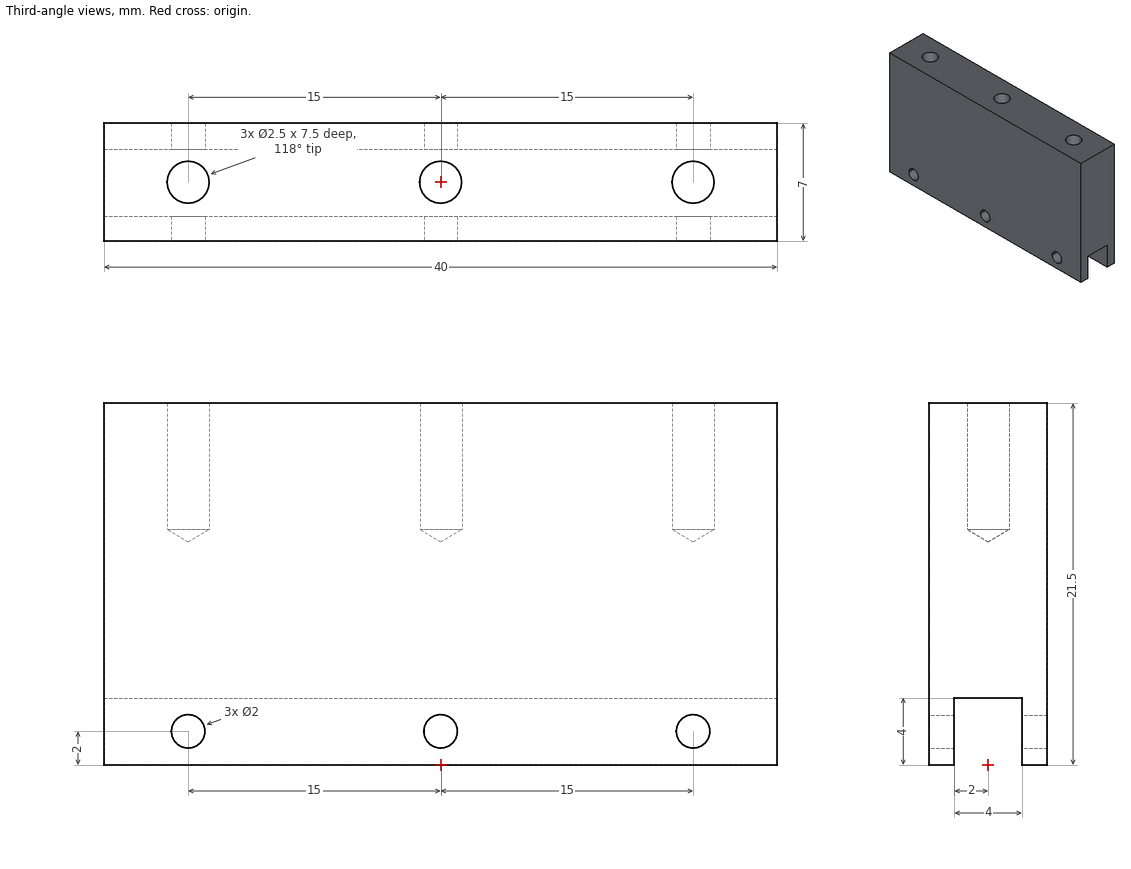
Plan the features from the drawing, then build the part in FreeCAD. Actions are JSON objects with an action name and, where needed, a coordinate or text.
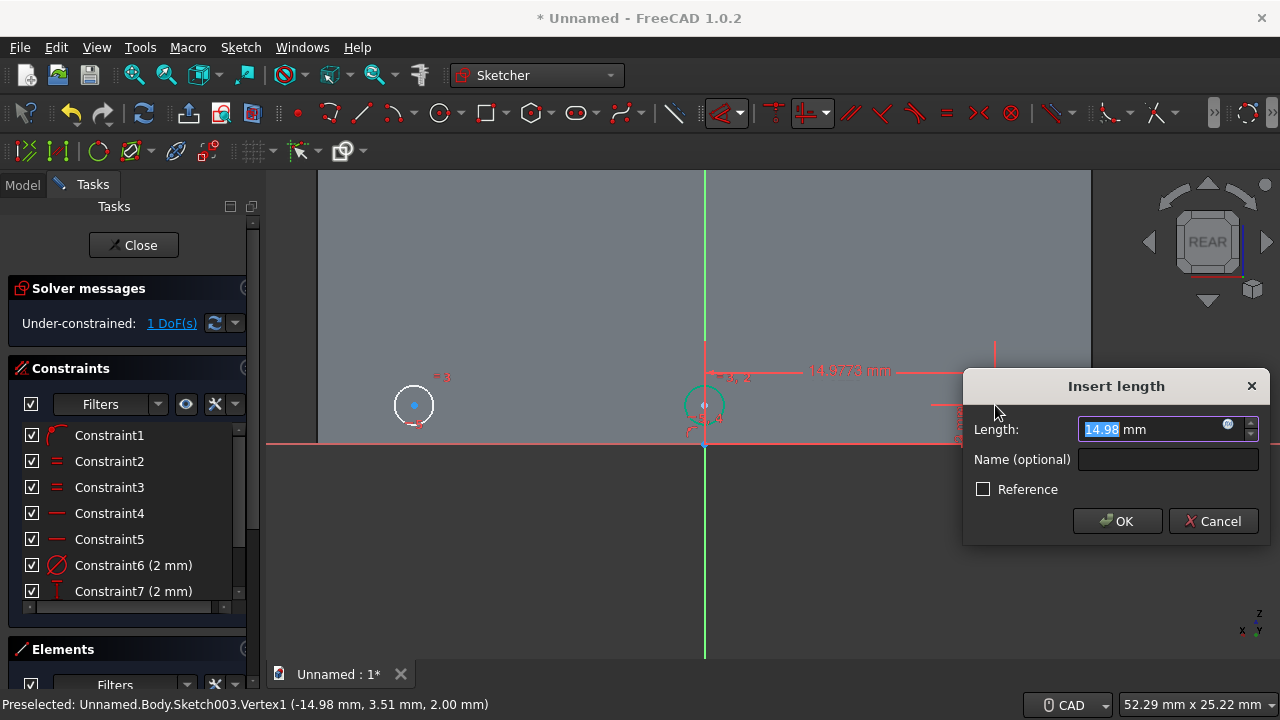
{"action": "type", "text": "15"}
{"action": "key", "text": "Return"}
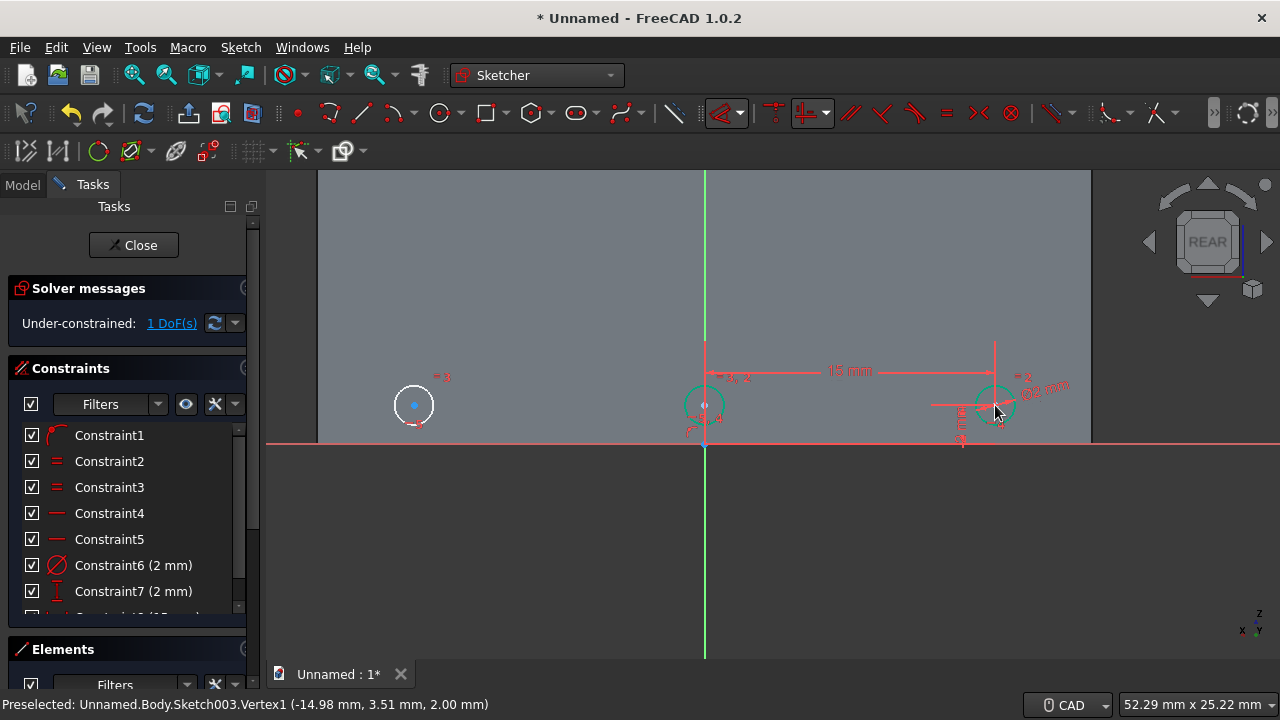
{"action": "left_click", "coordinate": [414, 405]}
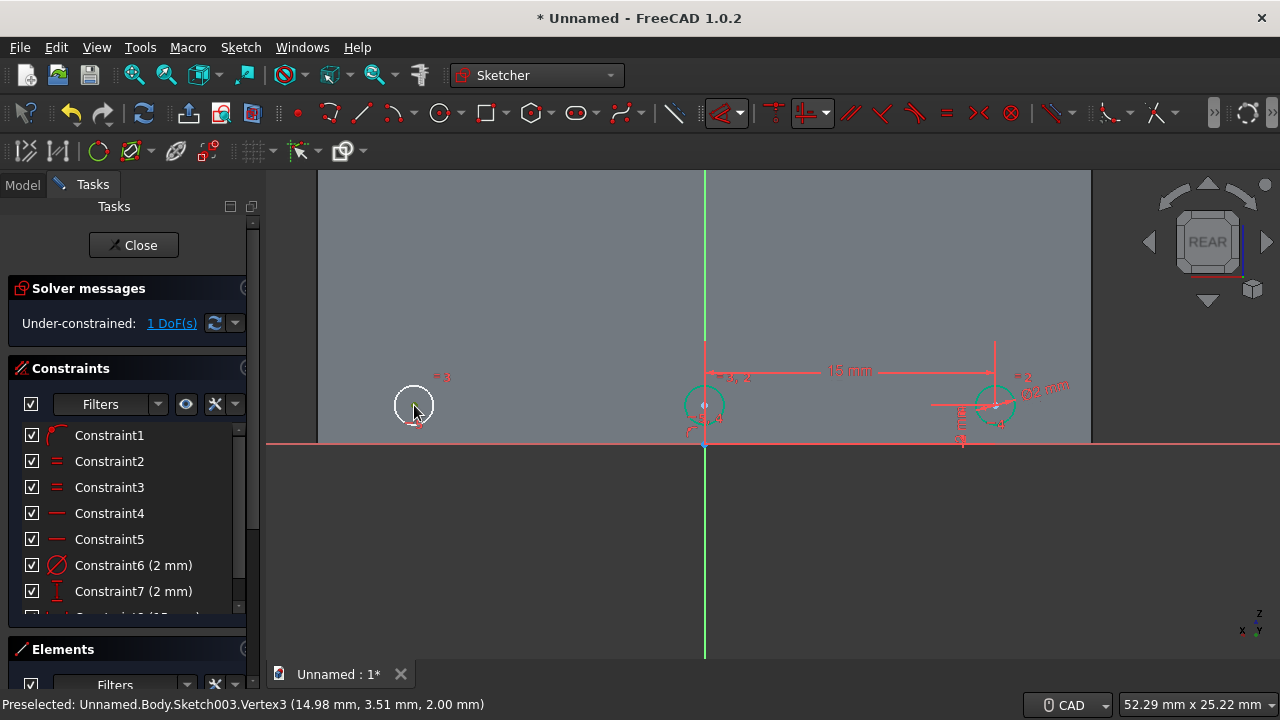
{"action": "left_click", "coordinate": [742, 114]}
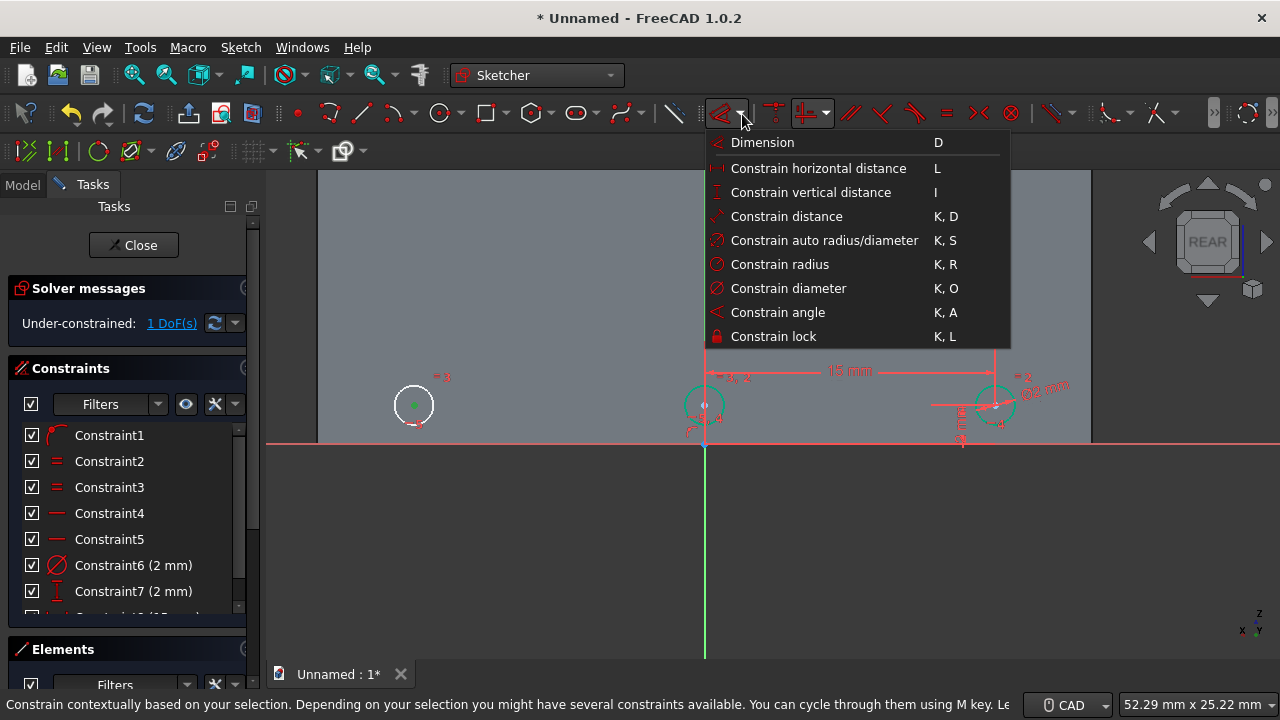
{"action": "left_click", "coordinate": [858, 168]}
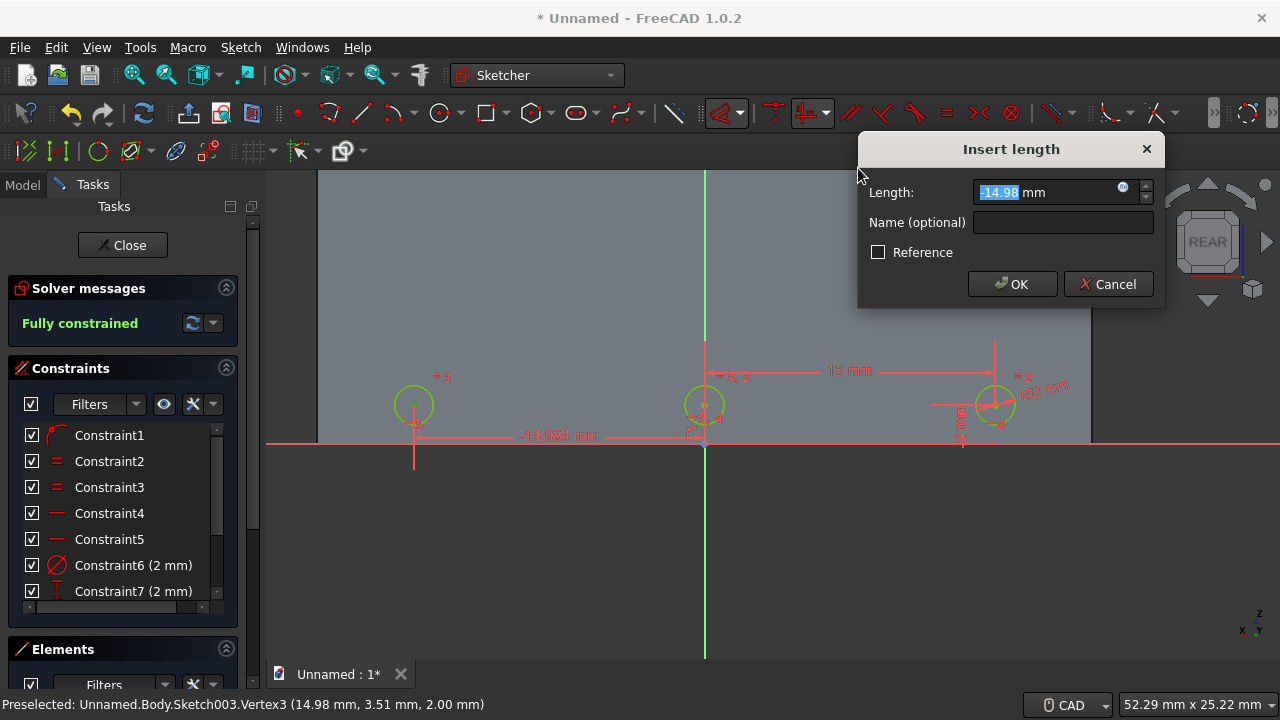
{"action": "type", "text": "-15"}
{"action": "key", "text": "Return"}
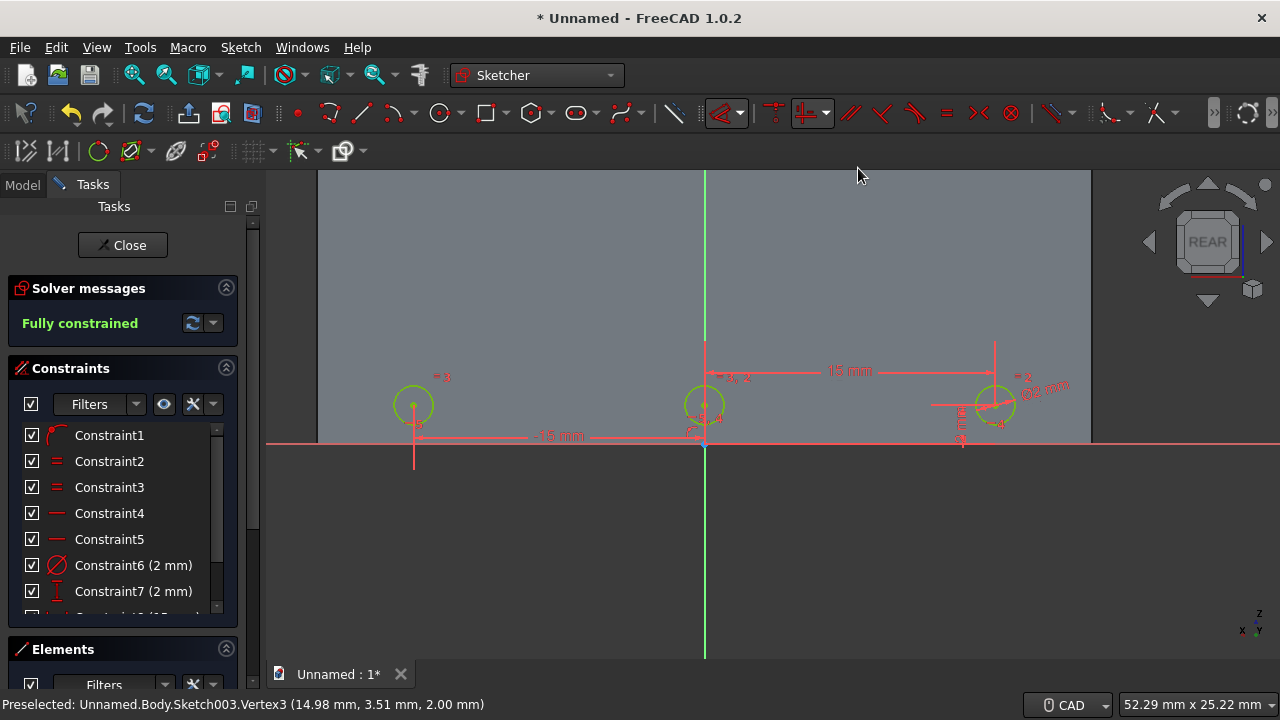
{"action": "left_click", "coordinate": [123, 245]}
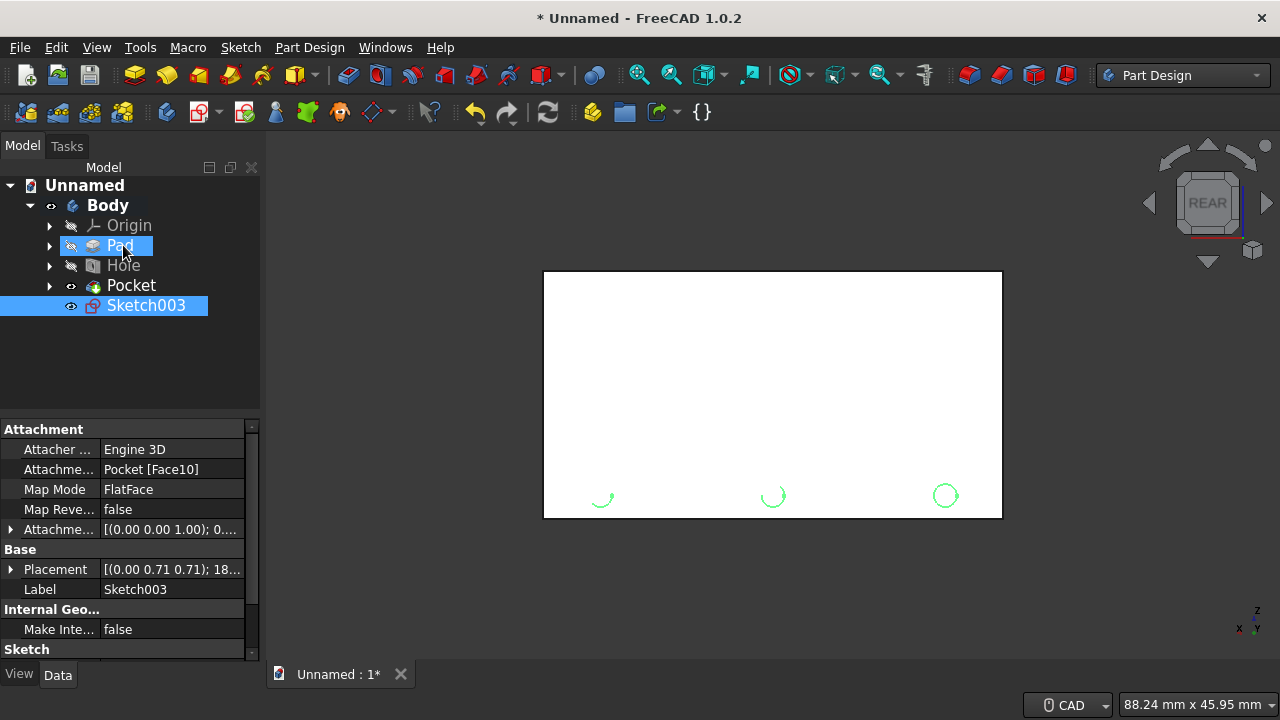
{"action": "left_click", "coordinate": [350, 76]}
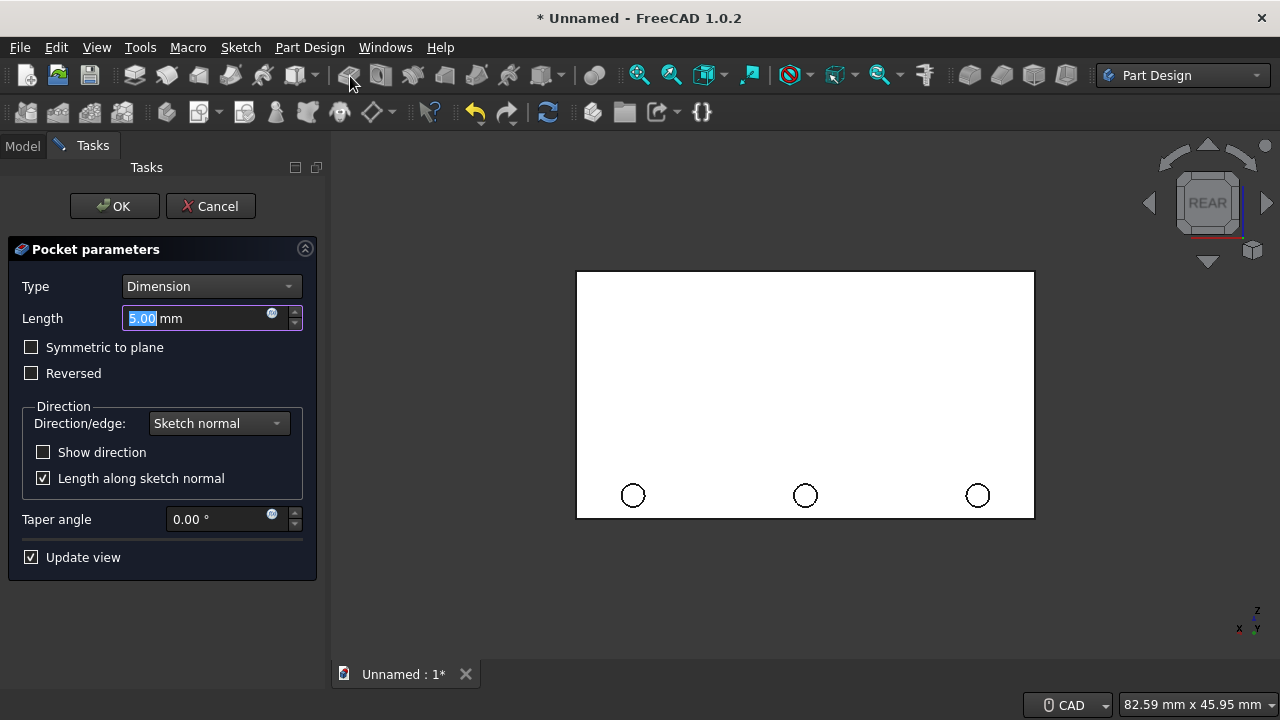
{"action": "left_click", "coordinate": [212, 286]}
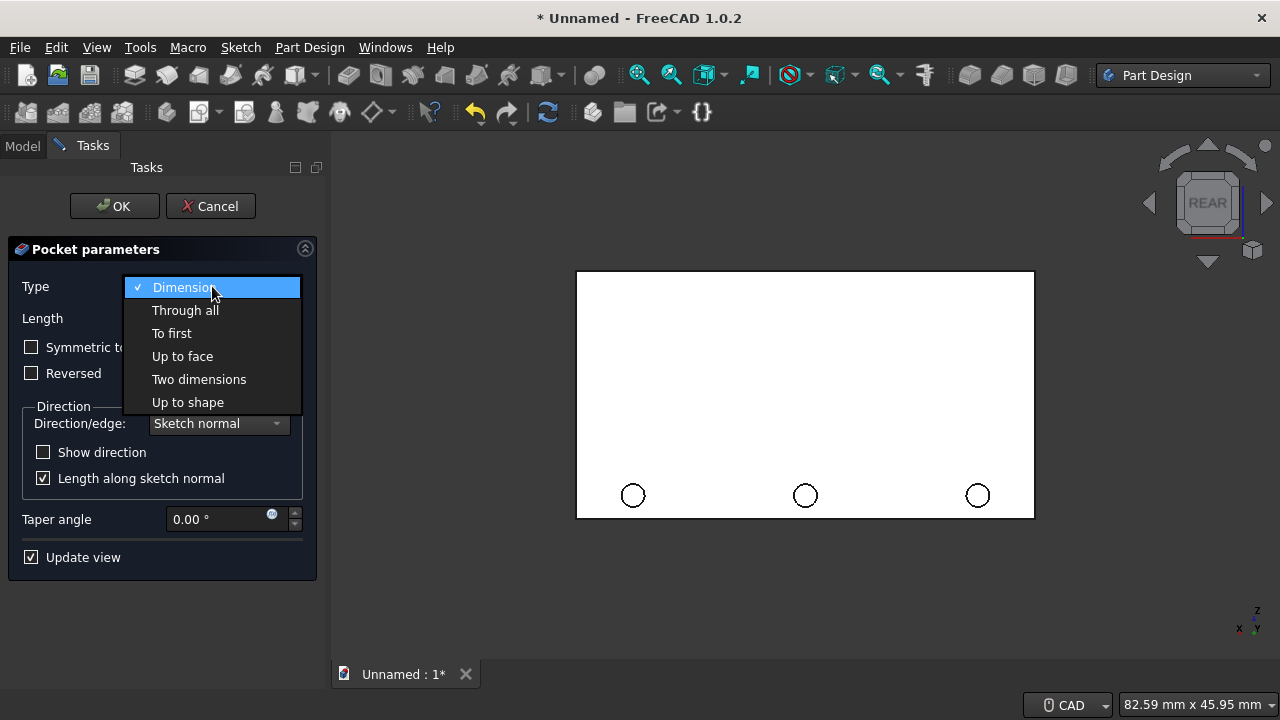
{"action": "left_click", "coordinate": [212, 310]}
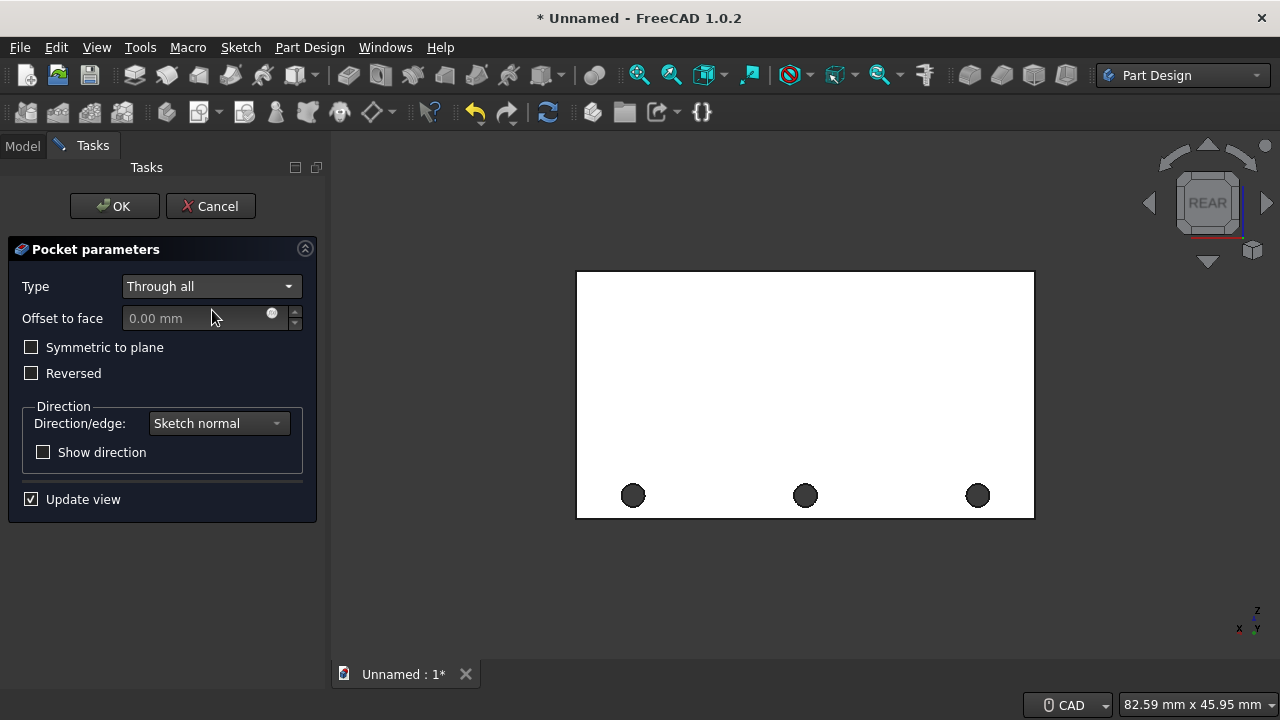
{"action": "left_click", "coordinate": [115, 206]}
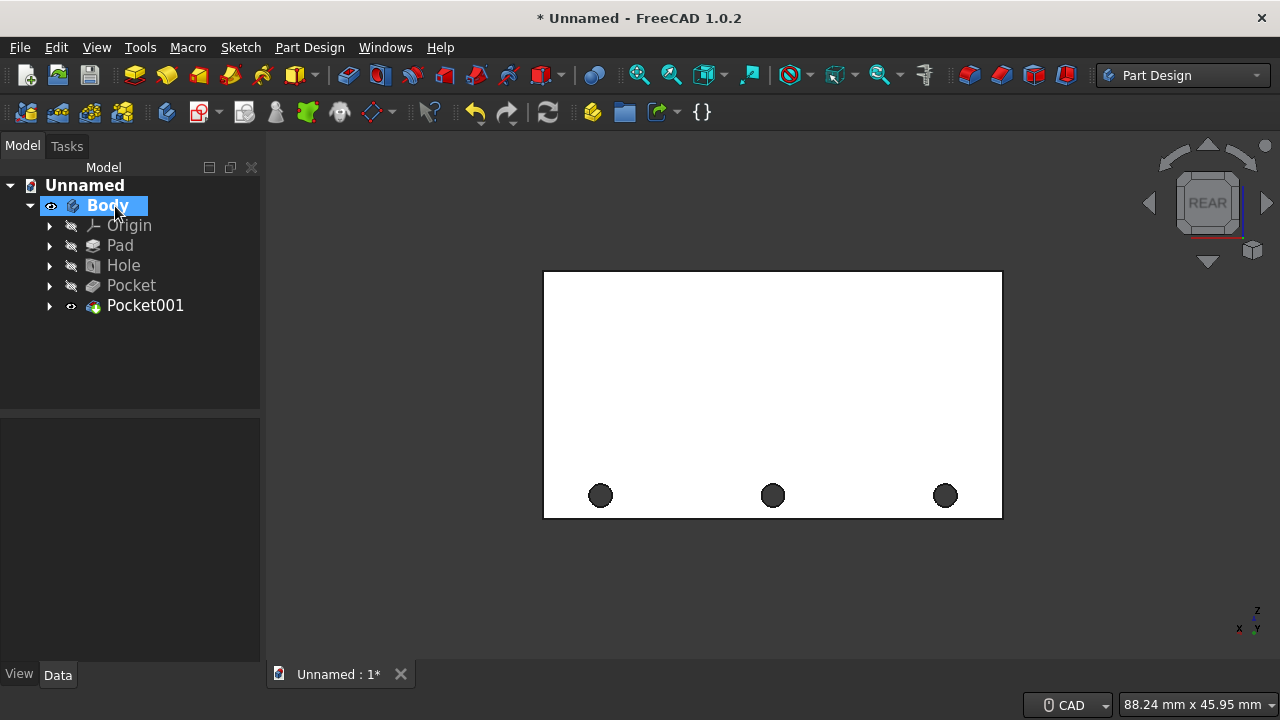
{"action": "key", "text": "0"}